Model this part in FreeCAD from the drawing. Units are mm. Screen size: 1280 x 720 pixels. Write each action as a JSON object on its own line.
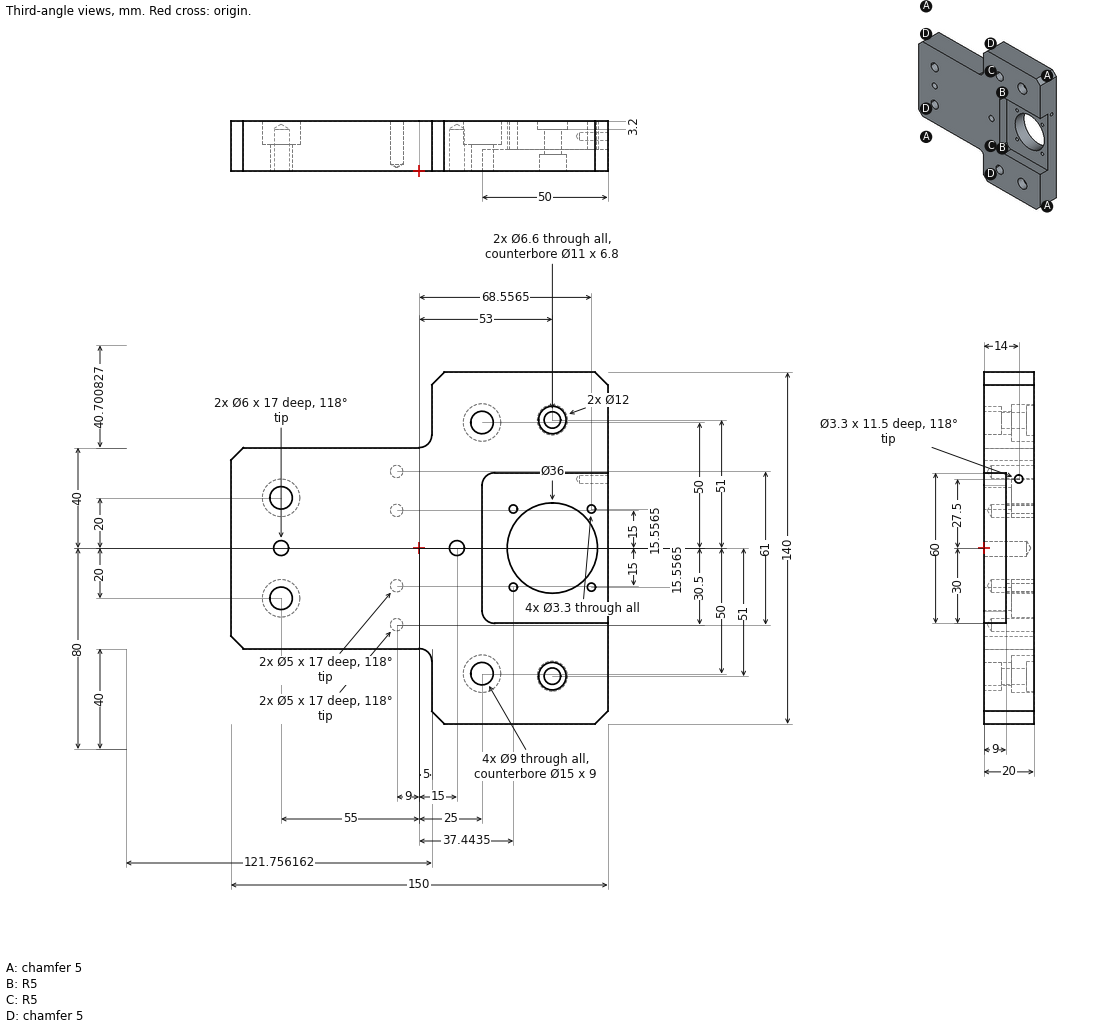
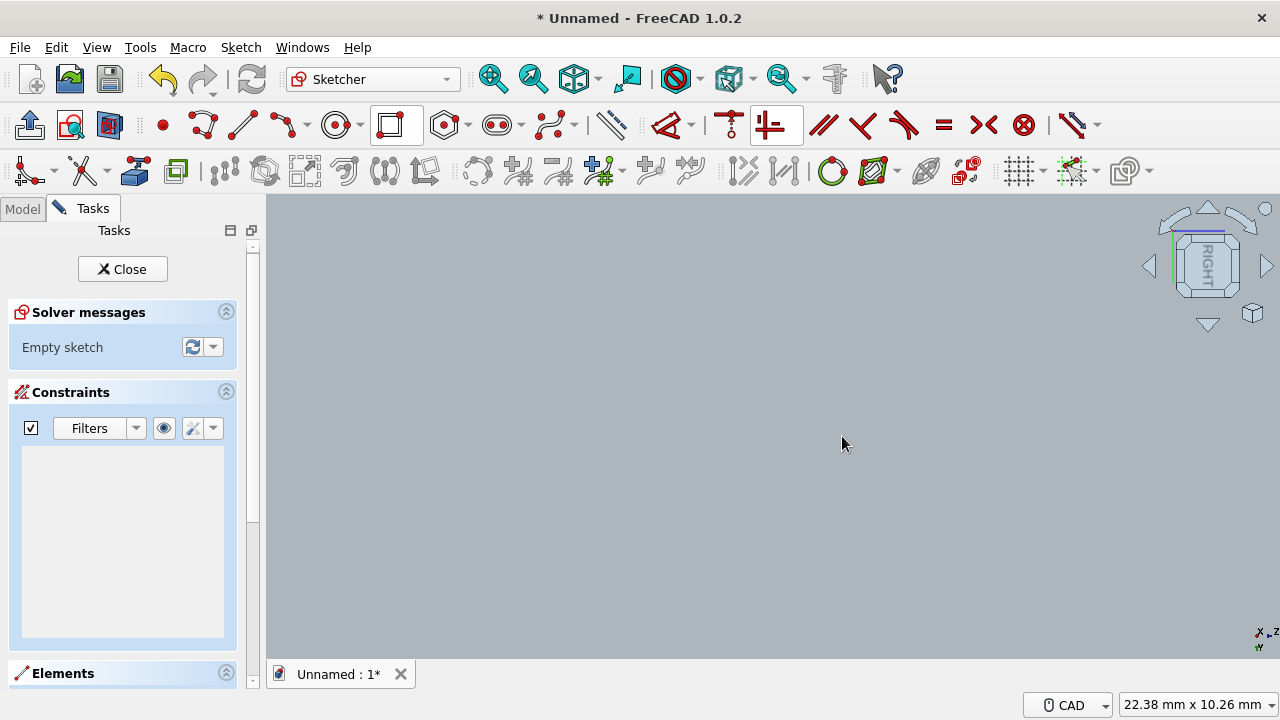
{"action": "scroll", "coordinate": [675, 404], "scroll_direction": "up", "scroll_amount": 3}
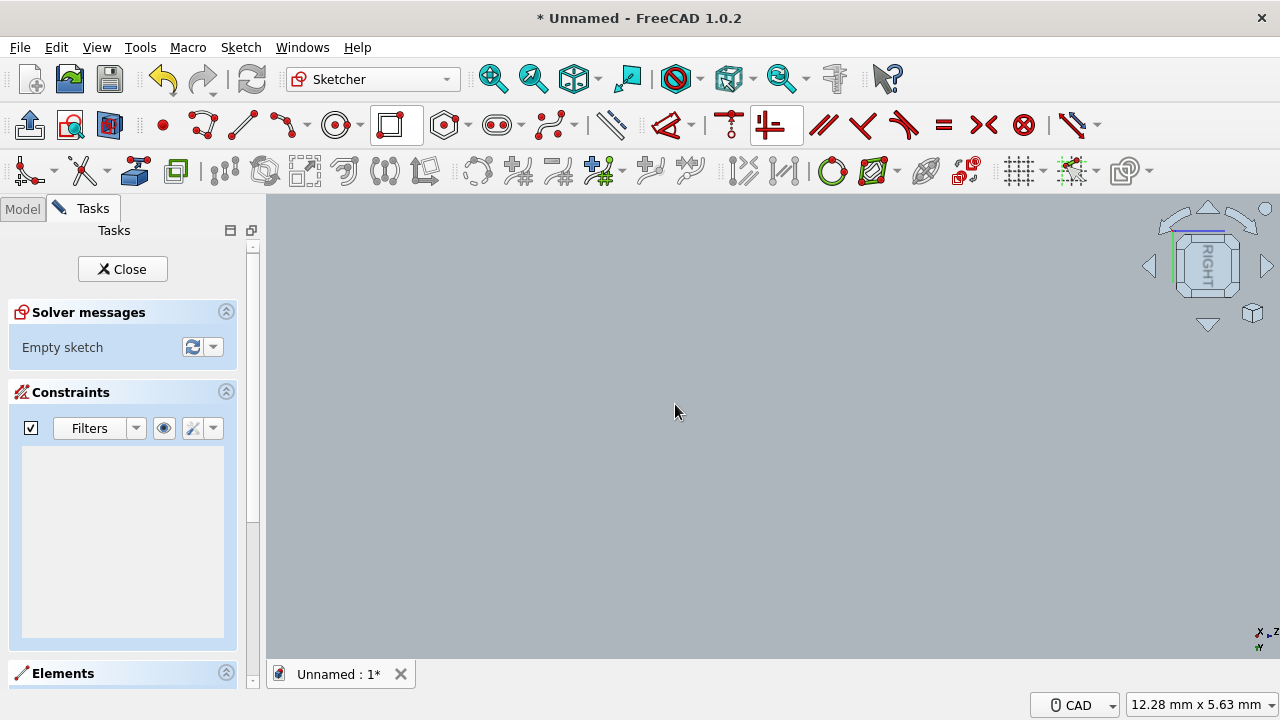
{"action": "left_click", "coordinate": [336, 126]}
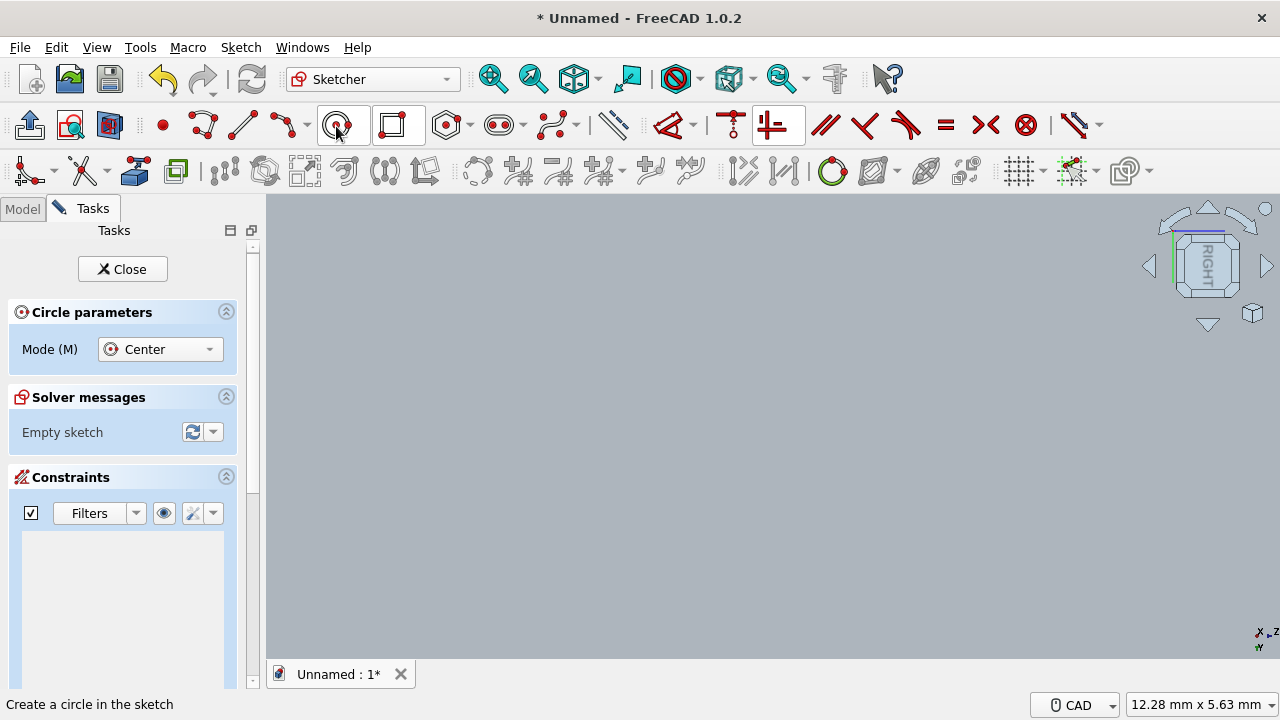
{"action": "left_click", "coordinate": [704, 426]}
{"action": "left_click", "coordinate": [800, 330]}
{"action": "key", "text": "Escape"}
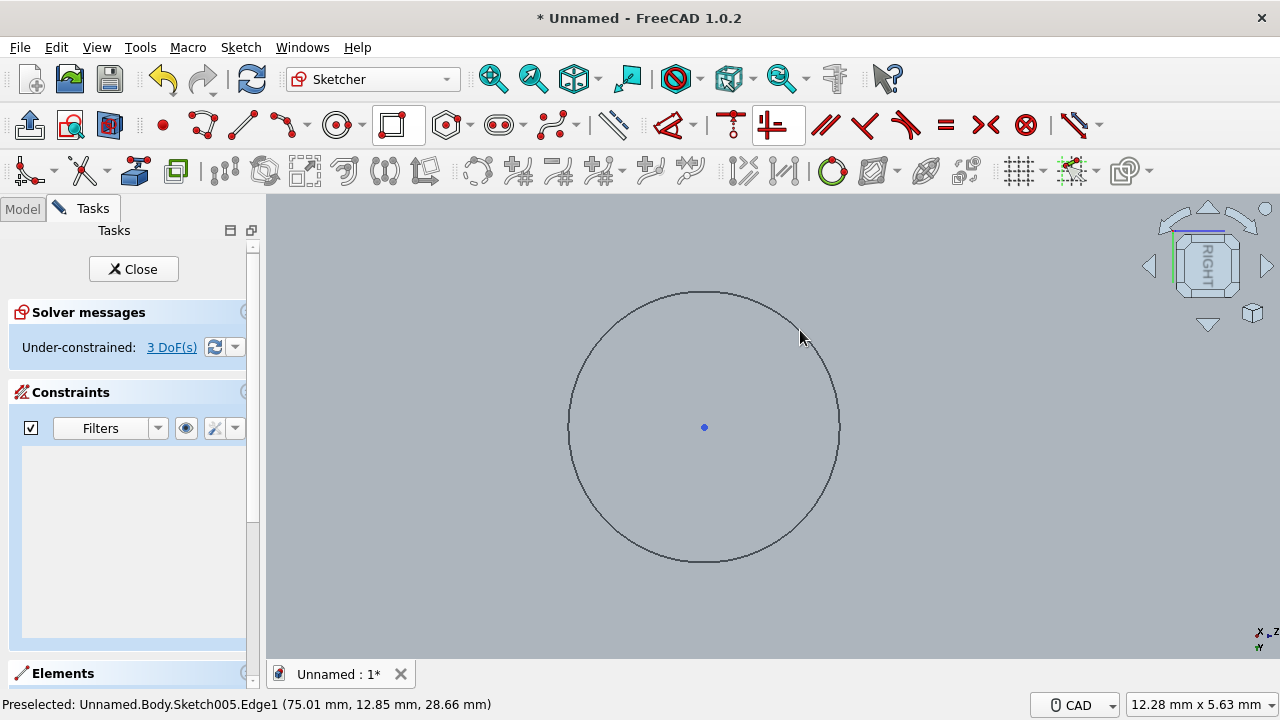
{"action": "left_click", "coordinate": [668, 126]}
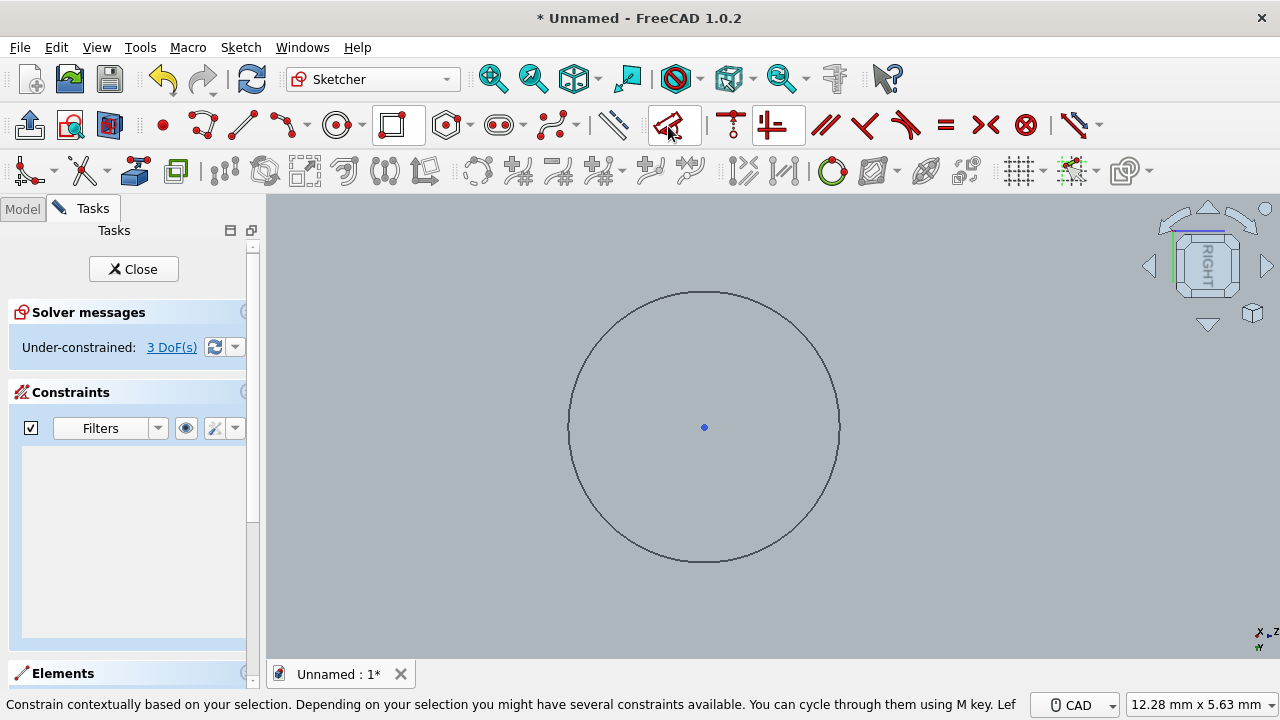
{"action": "left_click", "coordinate": [800, 331]}
{"action": "left_click", "coordinate": [823, 308]}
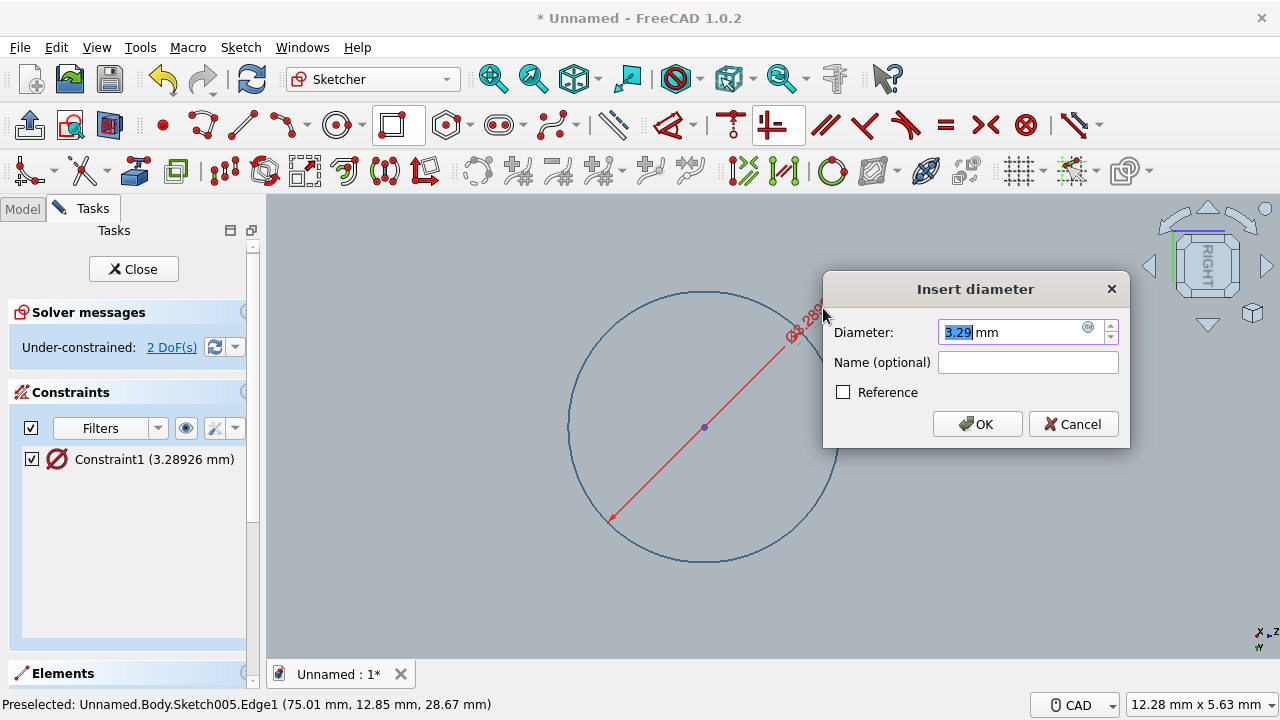
{"action": "type", "text": "3.3"}
{"action": "key", "text": "Return"}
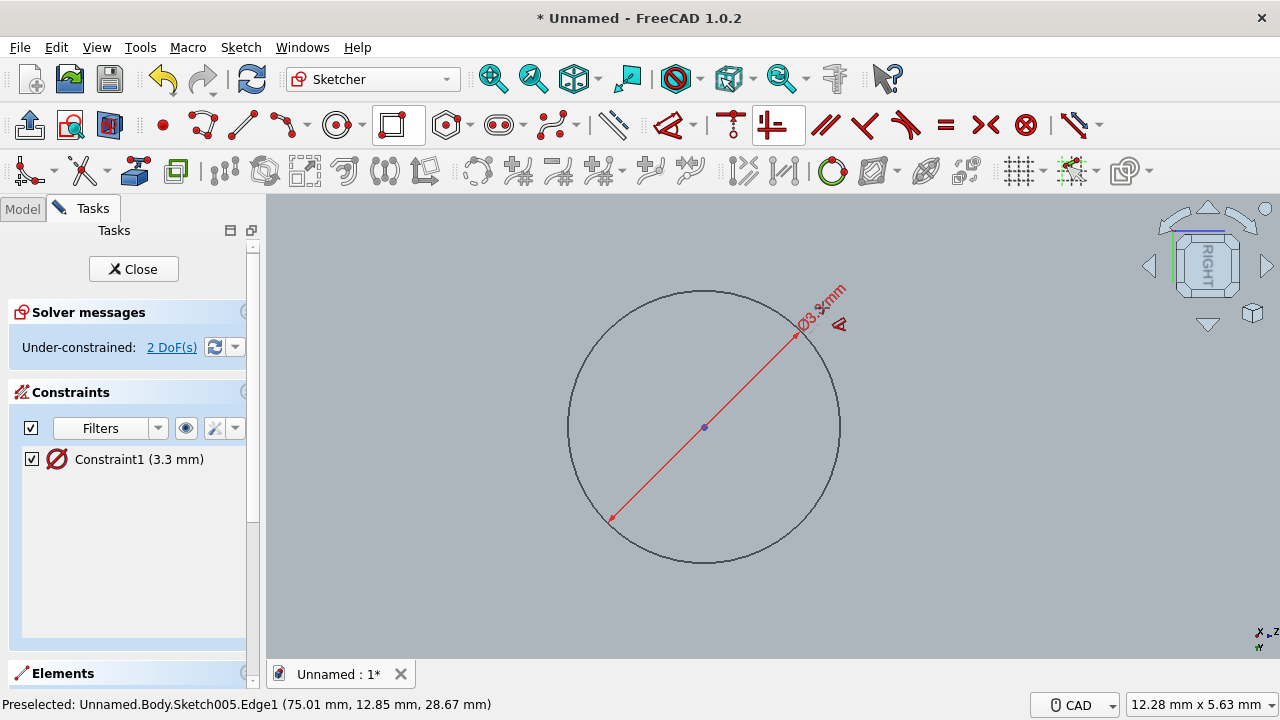
{"action": "left_click", "coordinate": [704, 427]}
{"action": "left_click", "coordinate": [738, 325]}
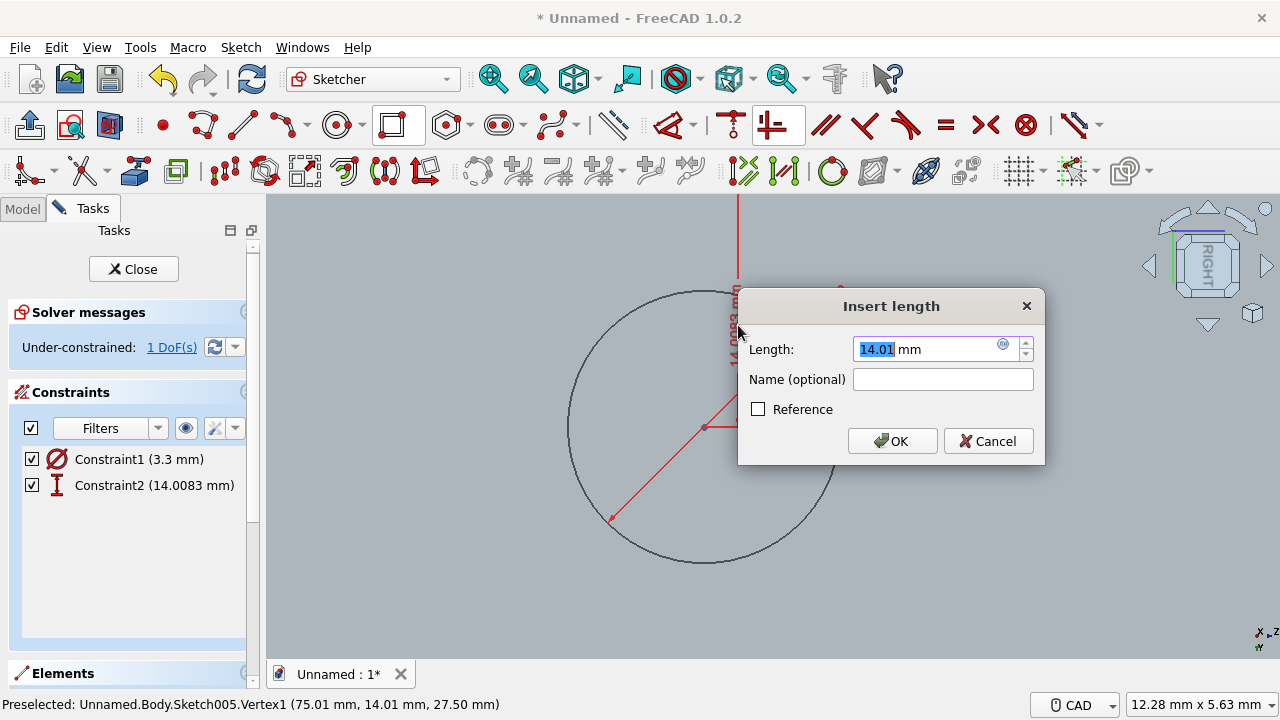
{"action": "type", "text": "14"}
{"action": "key", "text": "Return"}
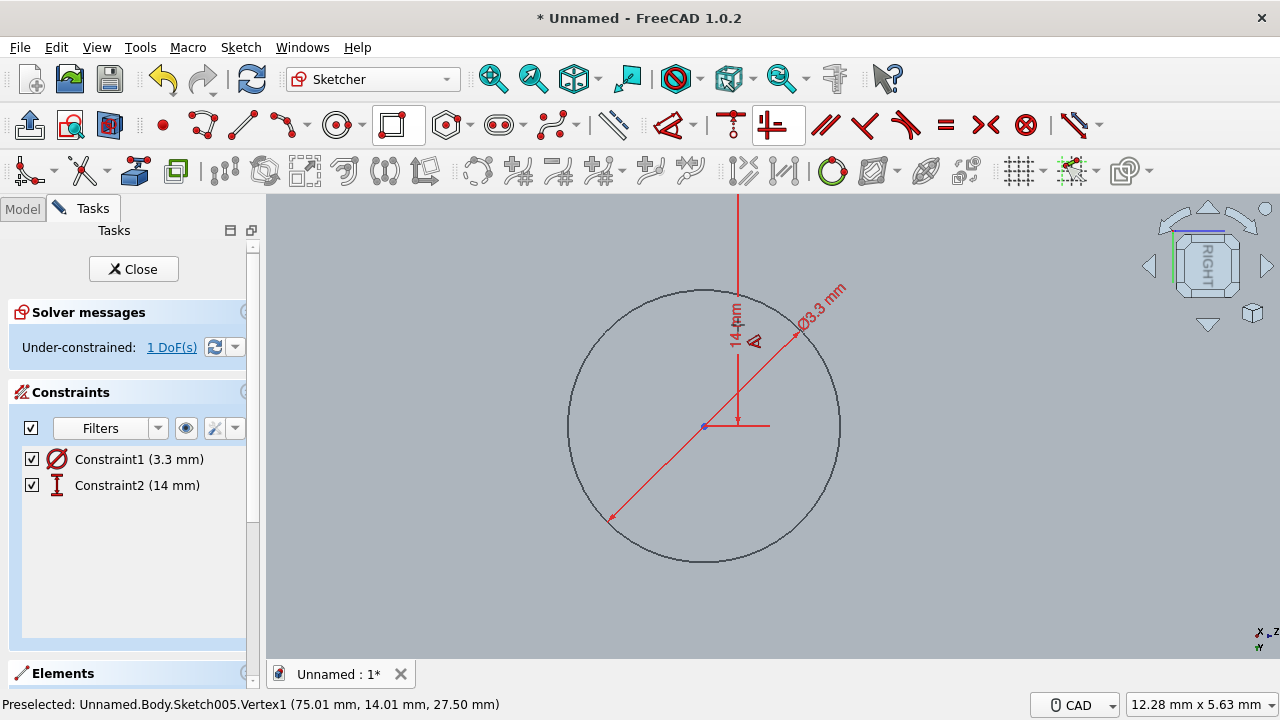
{"action": "left_click", "coordinate": [704, 426]}
{"action": "left_click", "coordinate": [499, 460]}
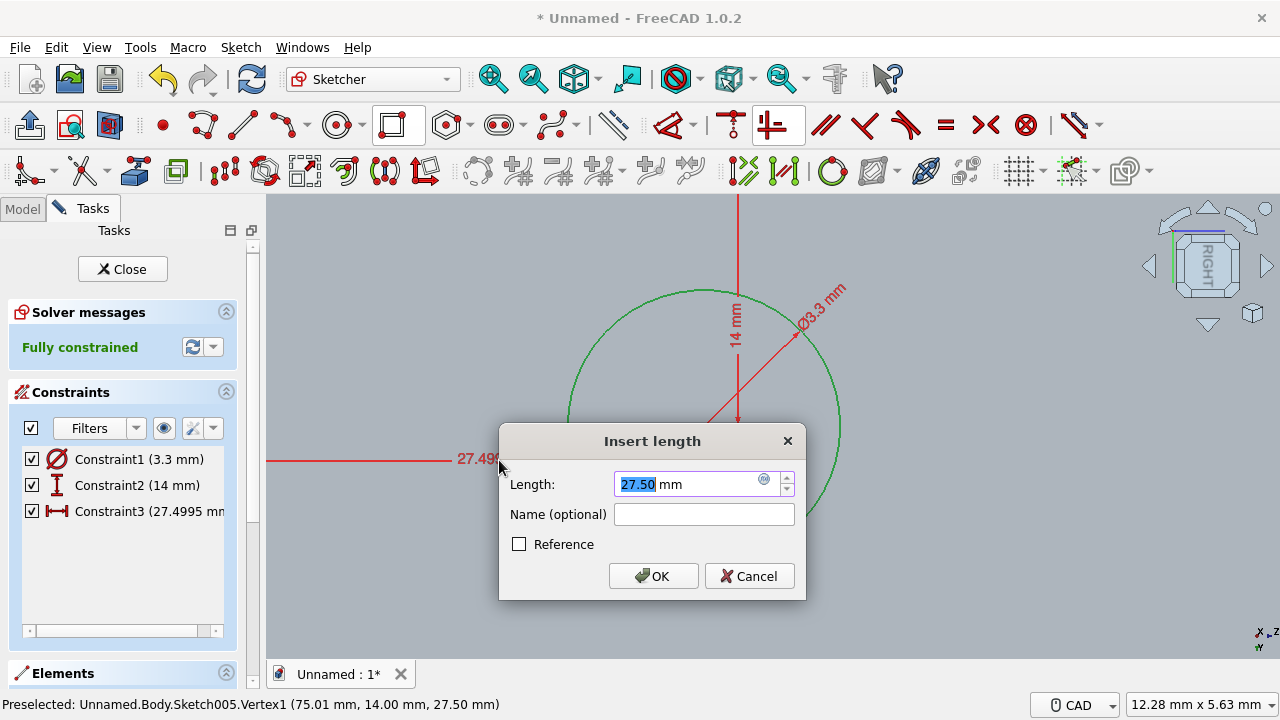
{"action": "type", "text": "27.5"}
{"action": "key", "text": "Return"}
{"action": "key", "text": "Escape"}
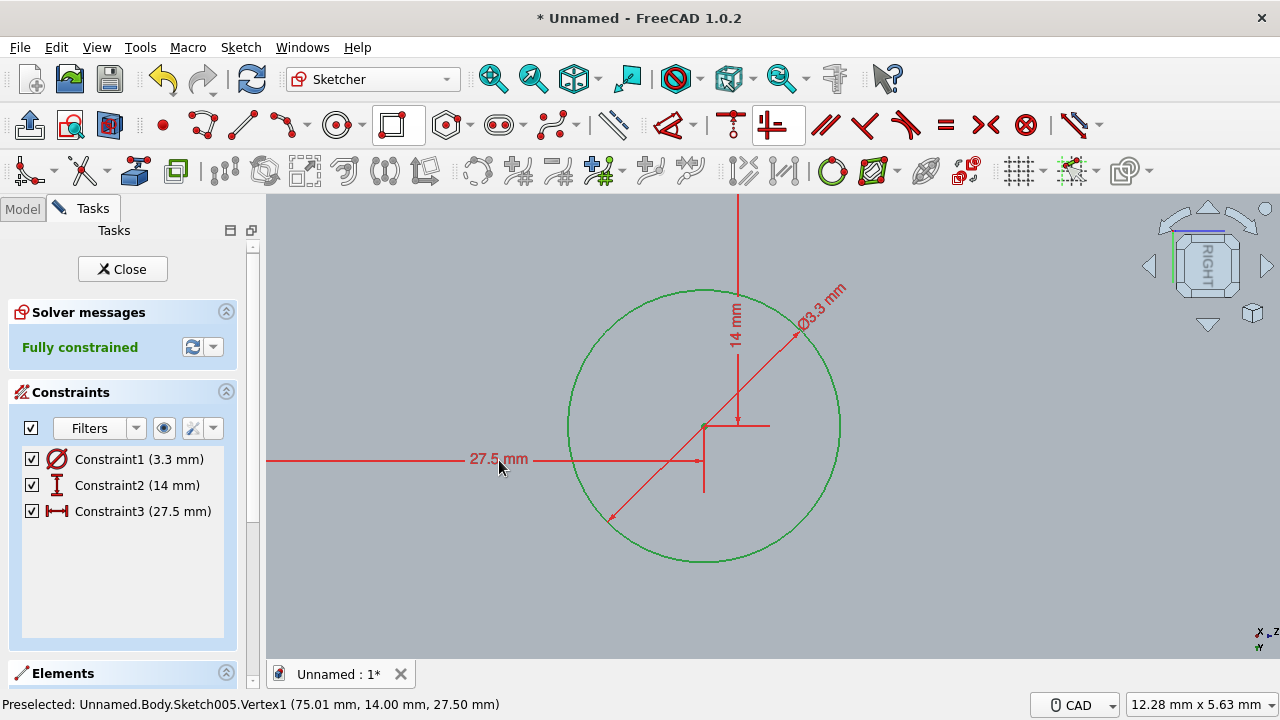
{"action": "left_click", "coordinate": [123, 269]}